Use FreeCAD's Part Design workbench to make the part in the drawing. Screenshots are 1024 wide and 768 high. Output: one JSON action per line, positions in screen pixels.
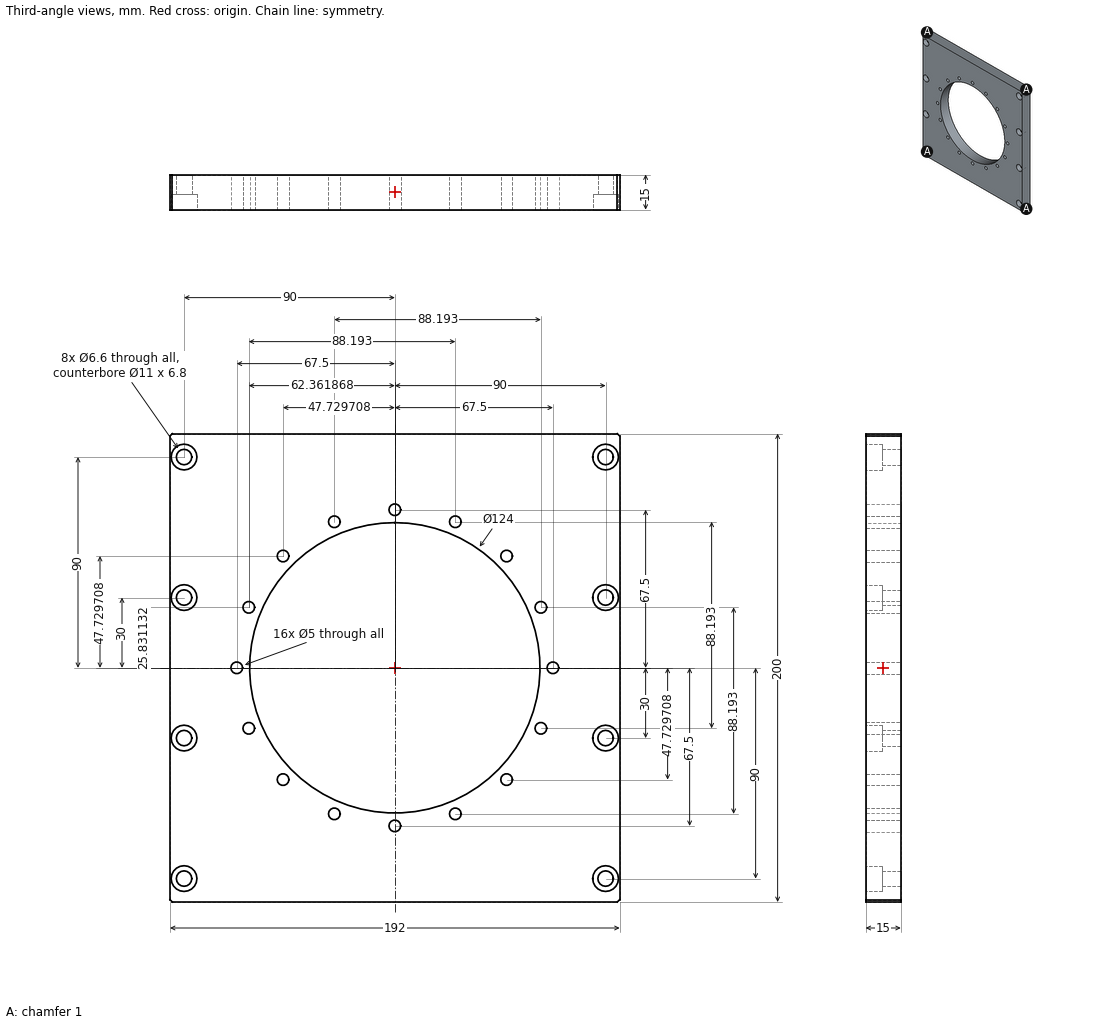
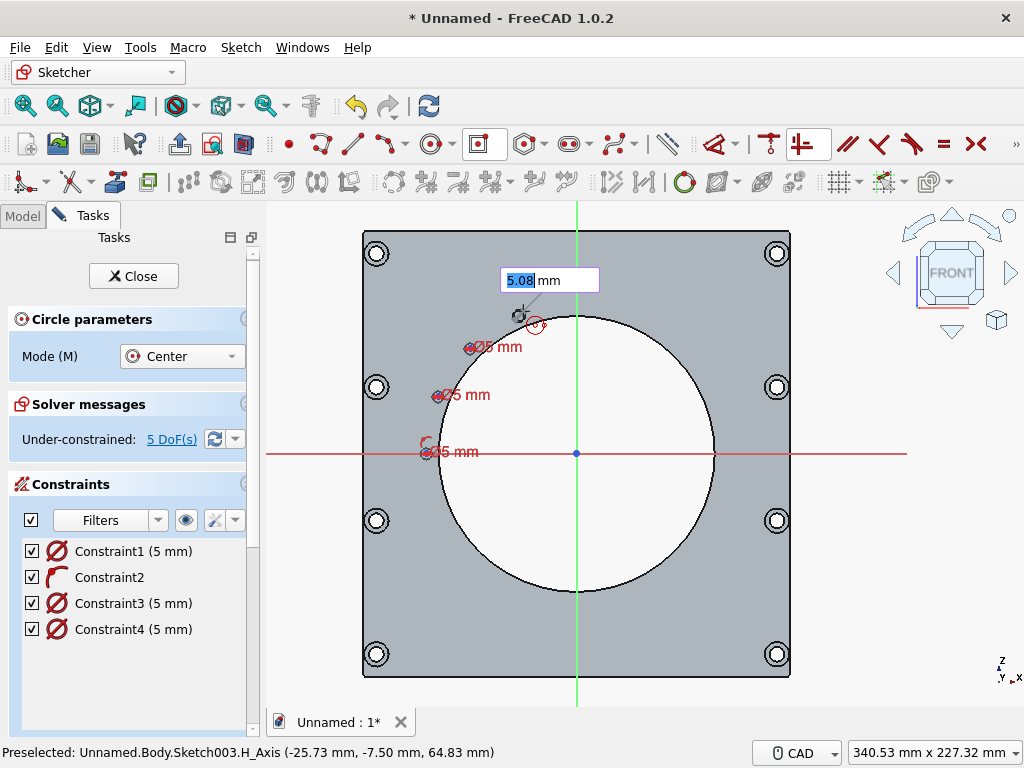
{"action": "type", "text": "5"}
{"action": "key", "text": "Return"}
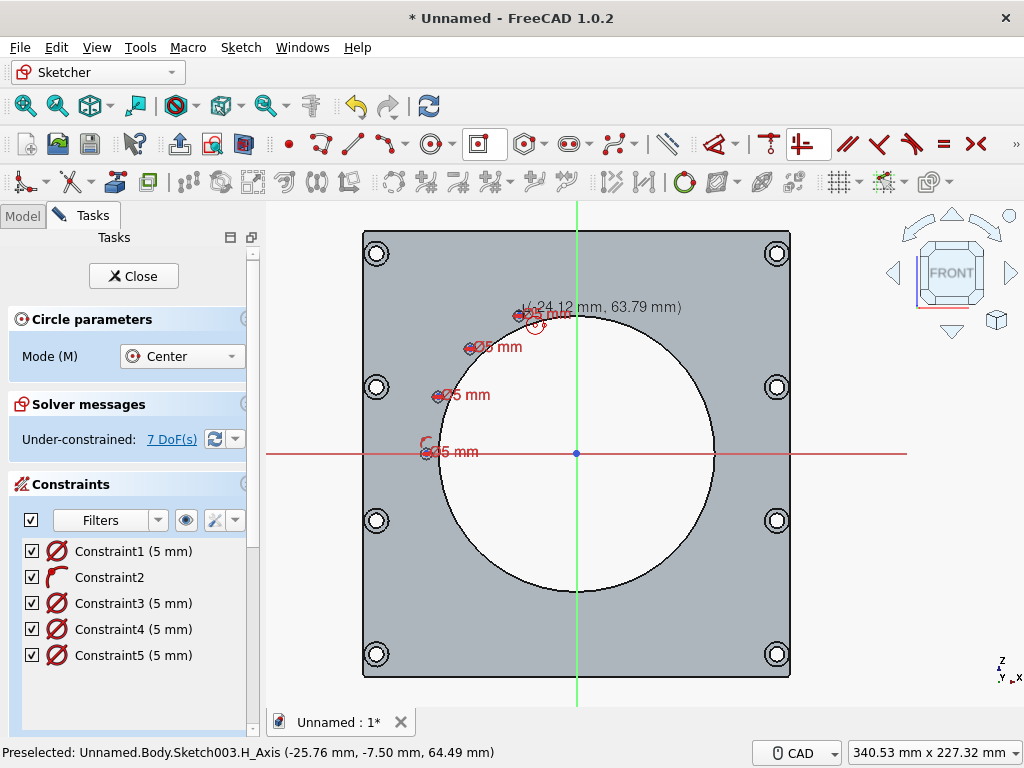
{"action": "scroll", "coordinate": [577, 304], "scroll_direction": "up", "scroll_amount": 8}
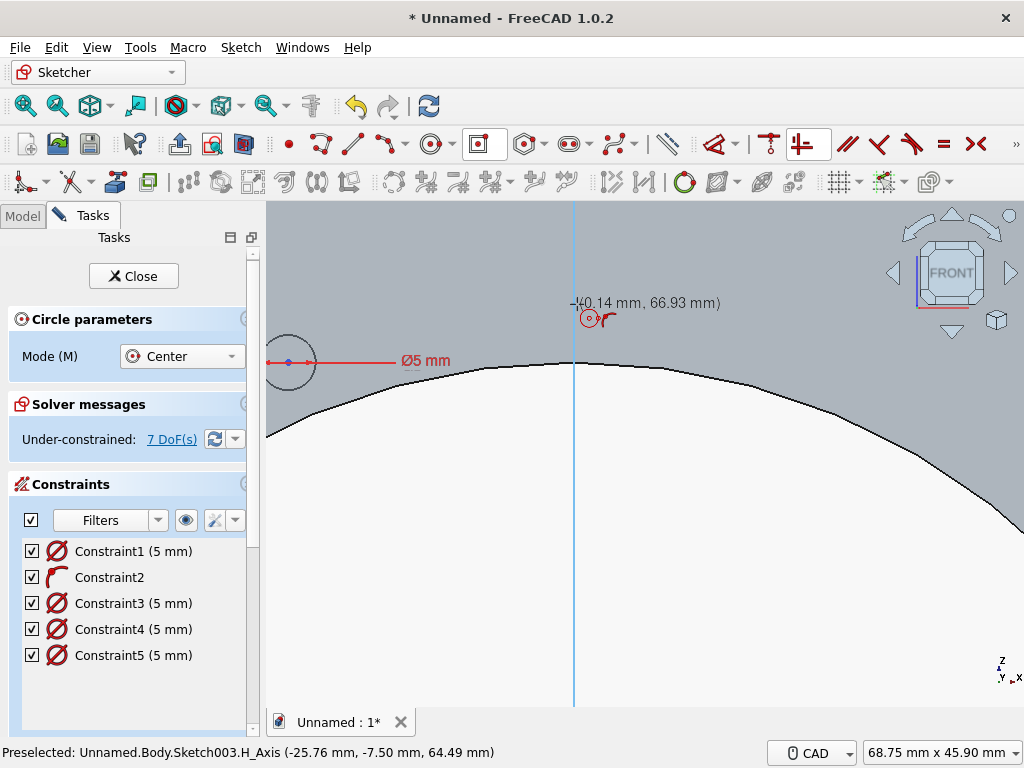
{"action": "scroll", "coordinate": [577, 304], "scroll_direction": "down", "scroll_amount": 8}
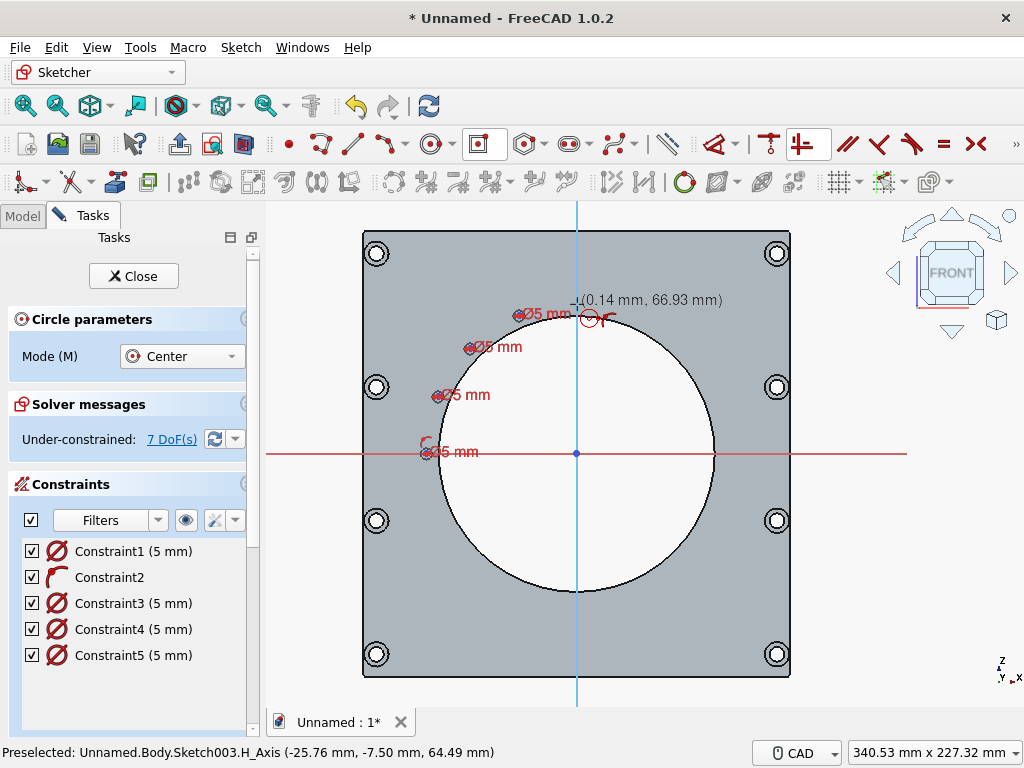
{"action": "left_click", "coordinate": [577, 304]}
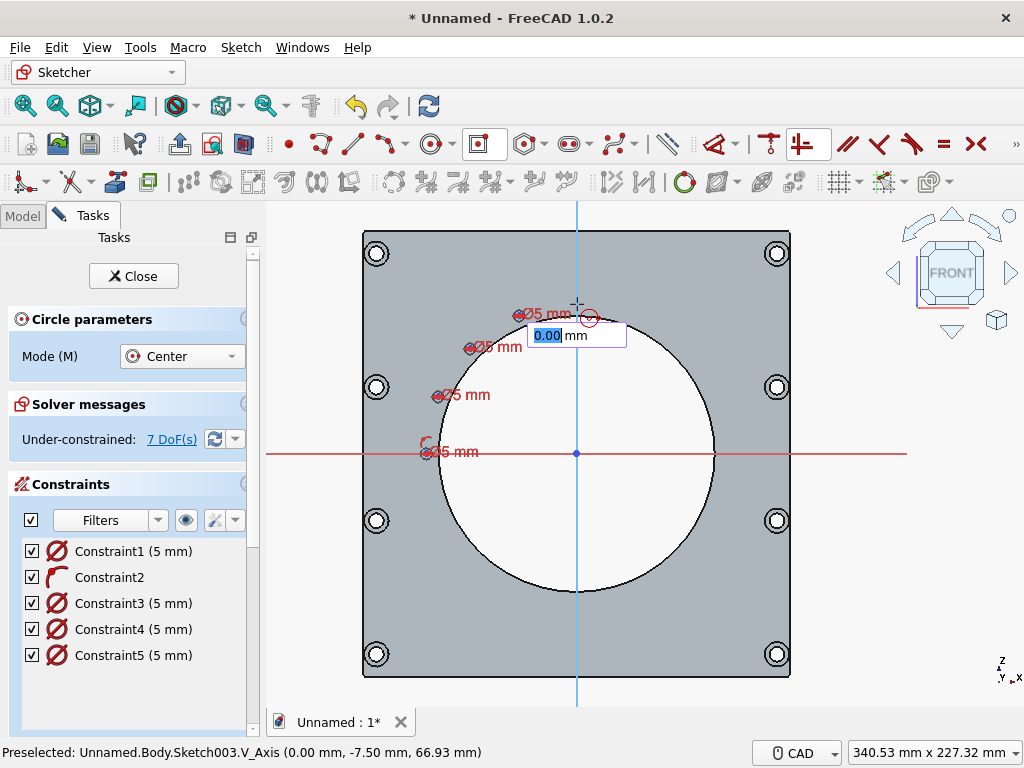
{"action": "scroll", "coordinate": [582, 302], "scroll_direction": "up", "scroll_amount": 6}
{"action": "mouse_move", "coordinate": [581, 301]}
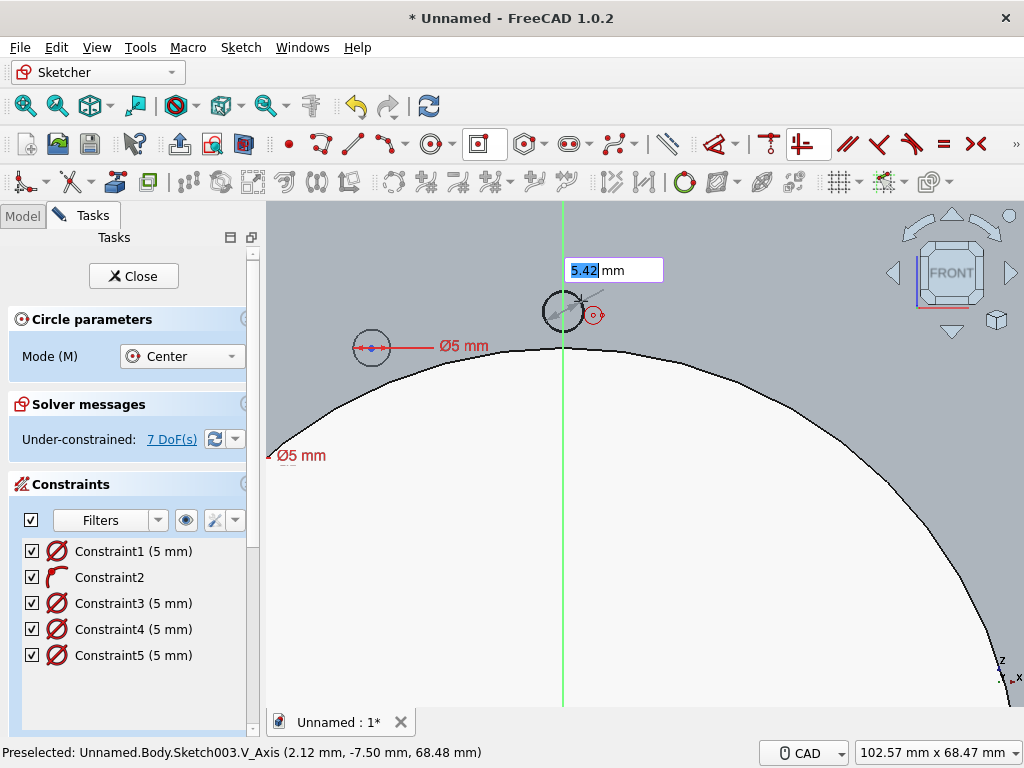
{"action": "type", "text": "5"}
{"action": "key", "text": "Return"}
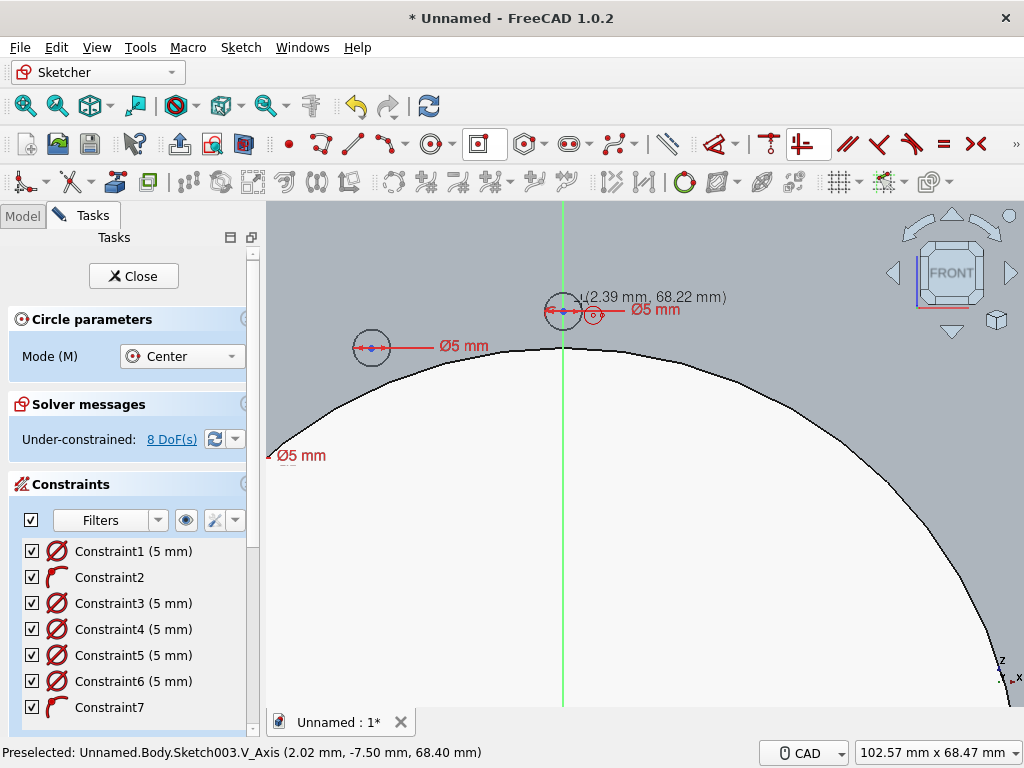
{"action": "scroll", "coordinate": [754, 345], "scroll_direction": "up", "scroll_amount": 2}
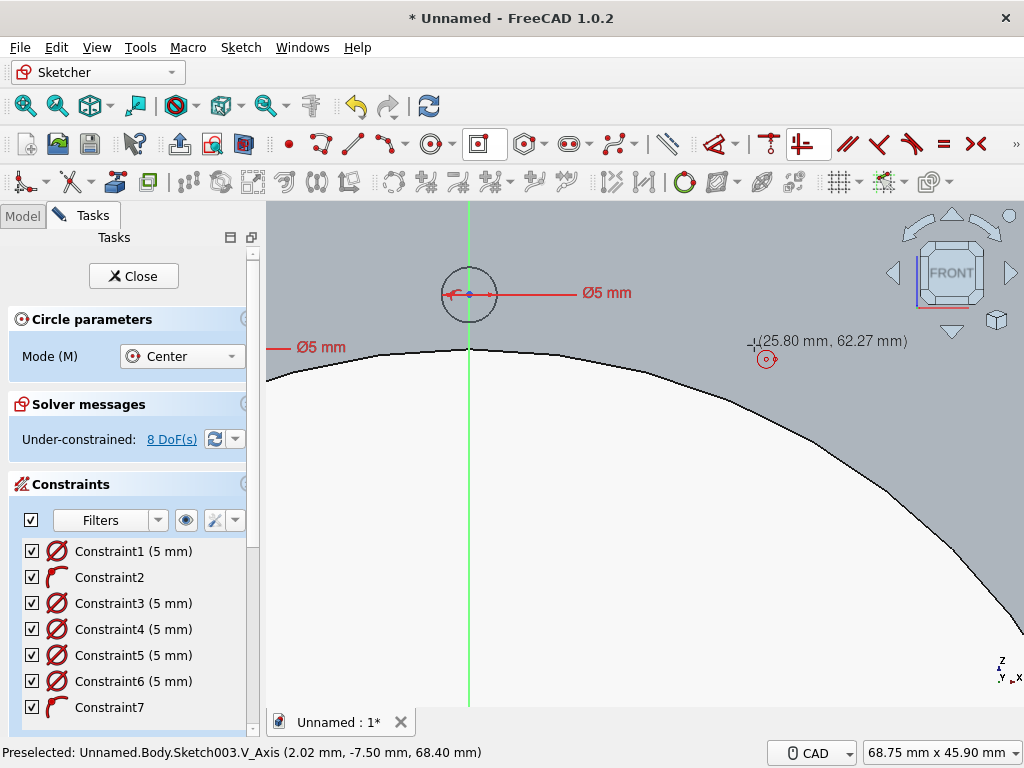
{"action": "scroll", "coordinate": [604, 308], "scroll_direction": "down", "scroll_amount": 8}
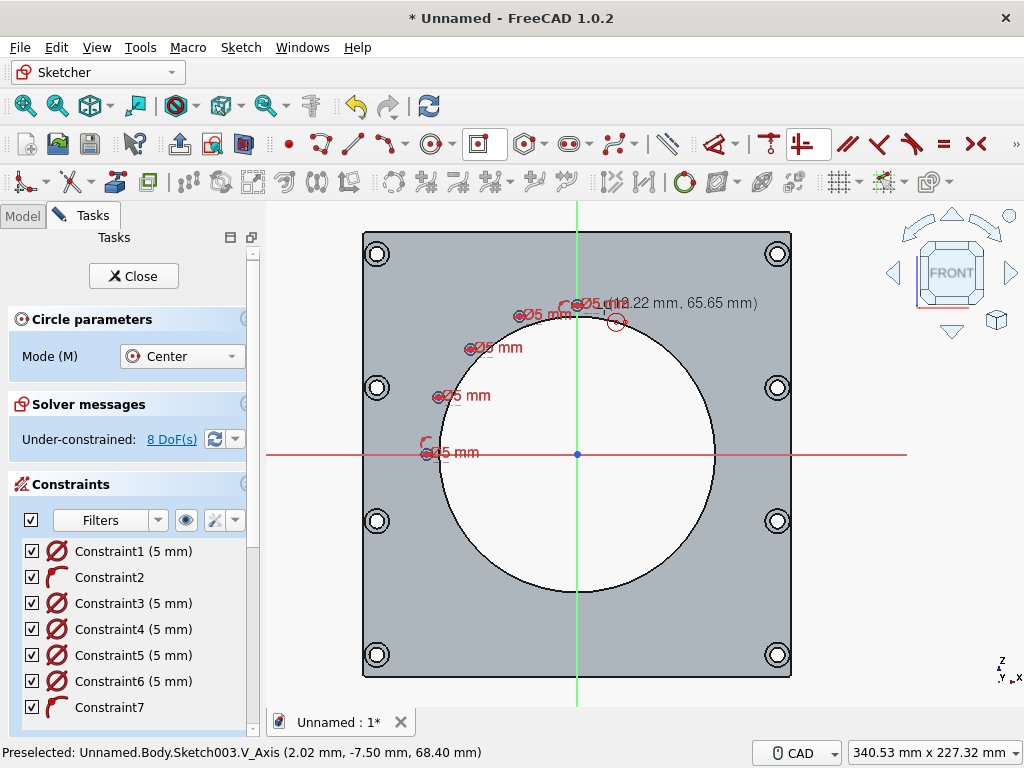
{"action": "left_click", "coordinate": [635, 316]}
{"action": "mouse_move", "coordinate": [639, 312]}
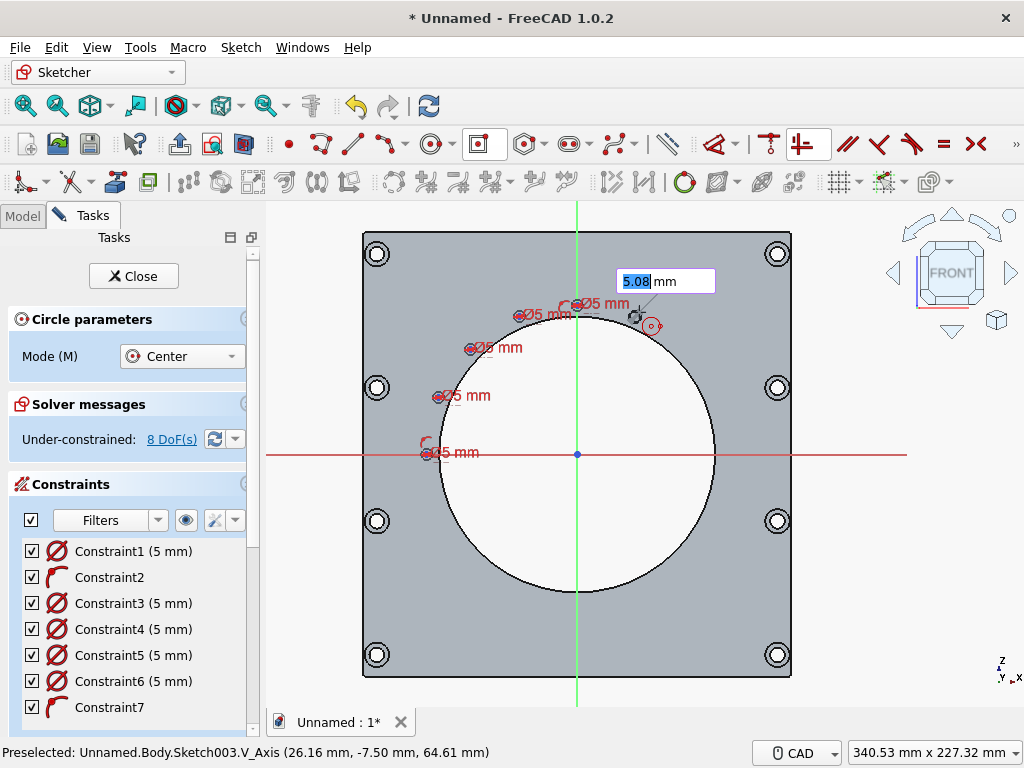
{"action": "type", "text": "5"}
{"action": "key", "text": "Return"}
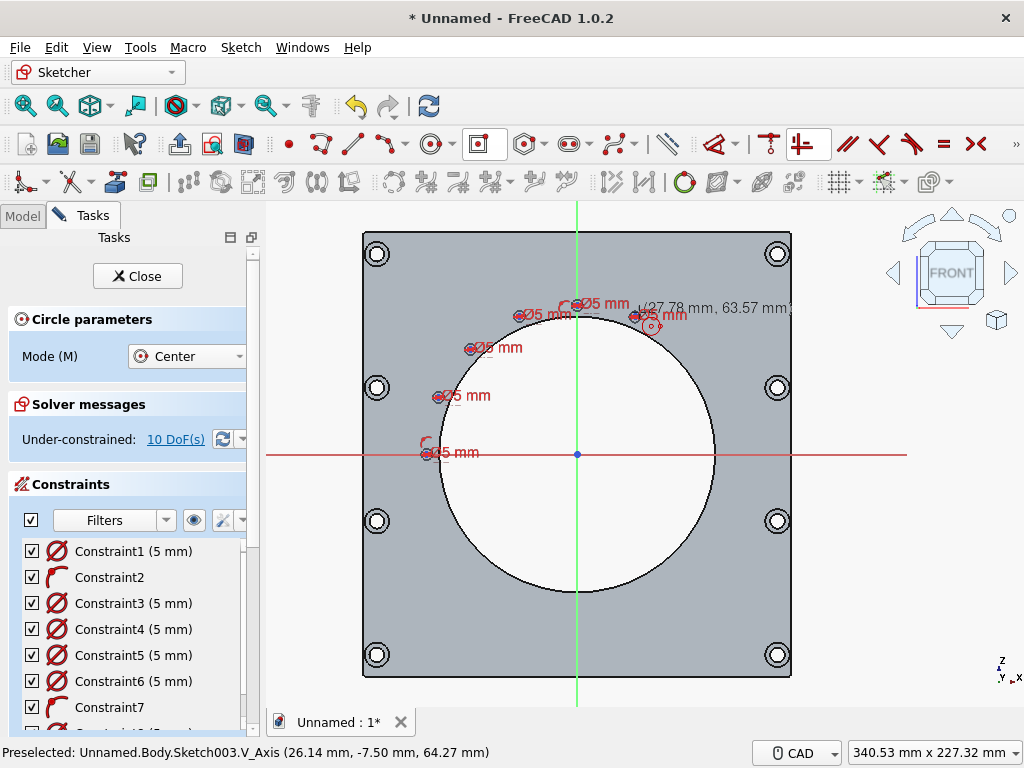
{"action": "scroll", "coordinate": [683, 348], "scroll_direction": "up", "scroll_amount": 8}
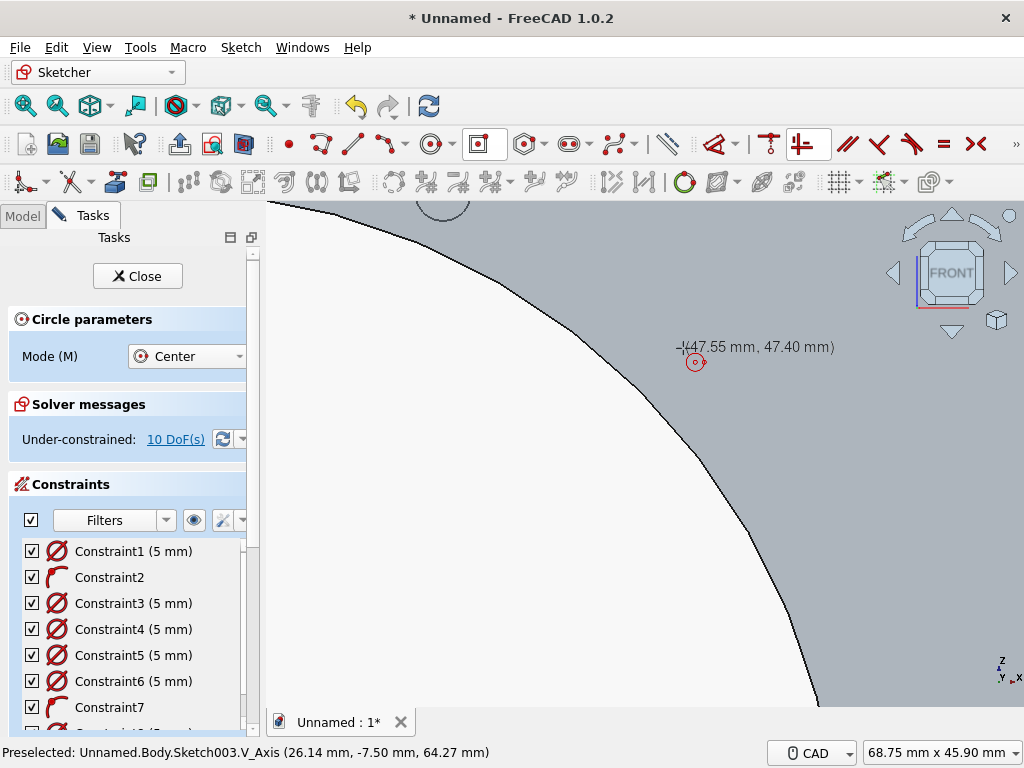
{"action": "scroll", "coordinate": [683, 348], "scroll_direction": "down", "scroll_amount": 8}